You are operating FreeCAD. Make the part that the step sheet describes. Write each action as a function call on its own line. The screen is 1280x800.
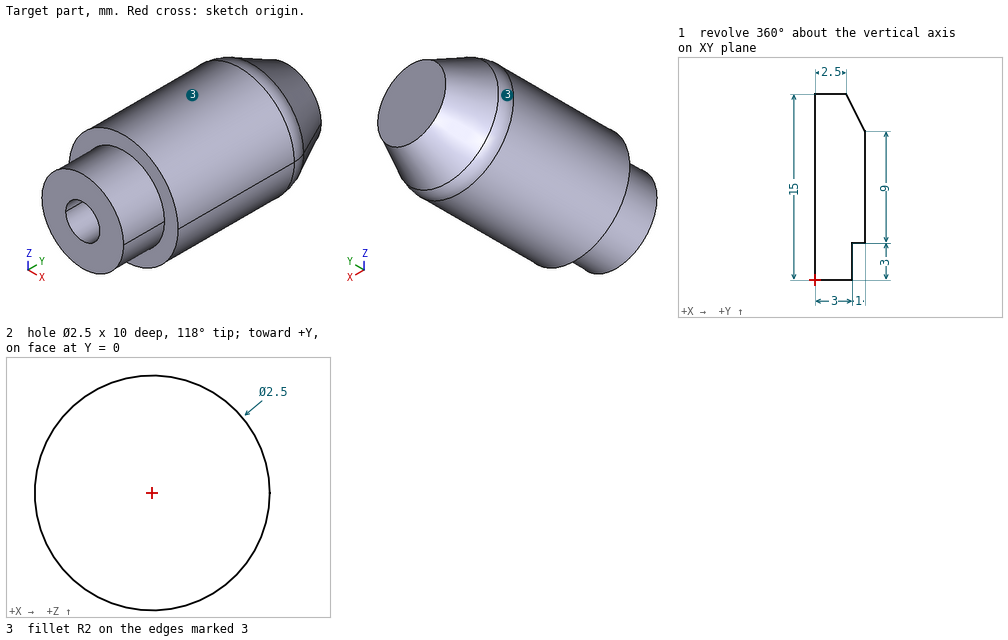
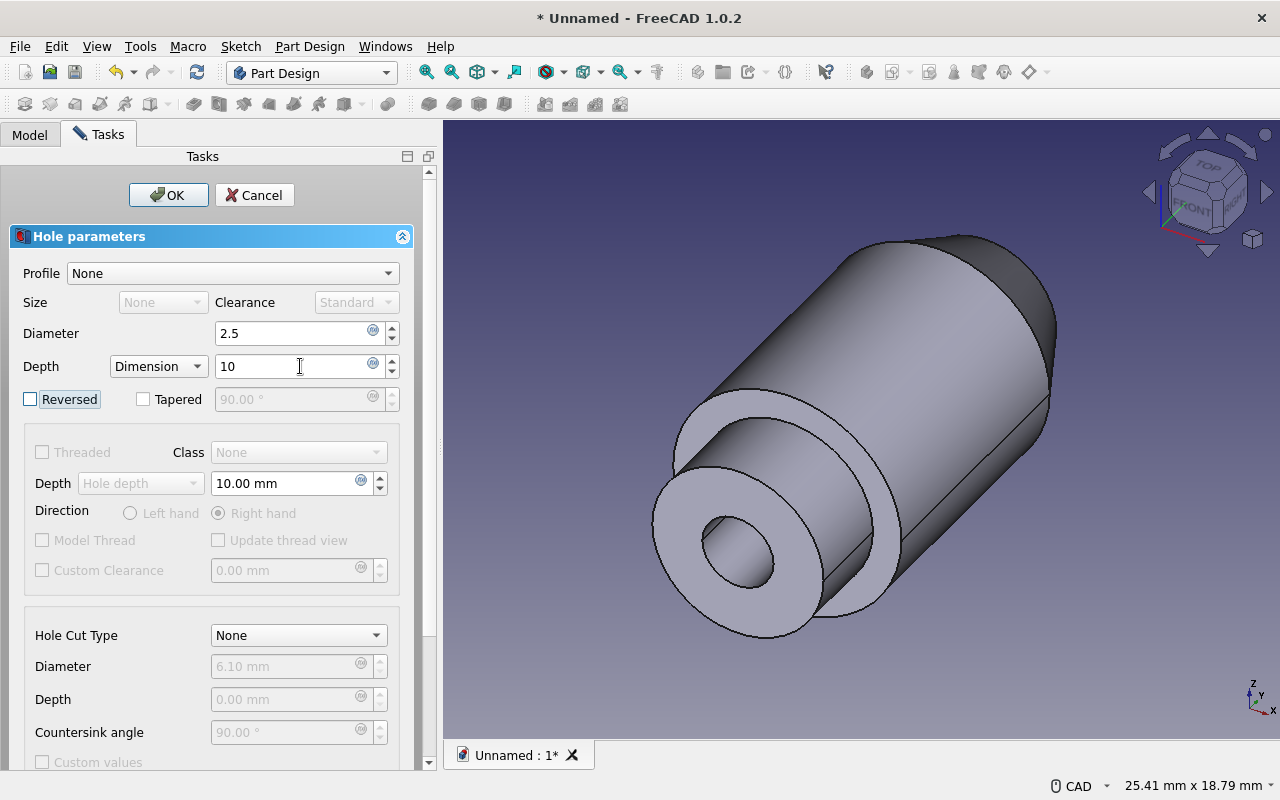
click(169, 195)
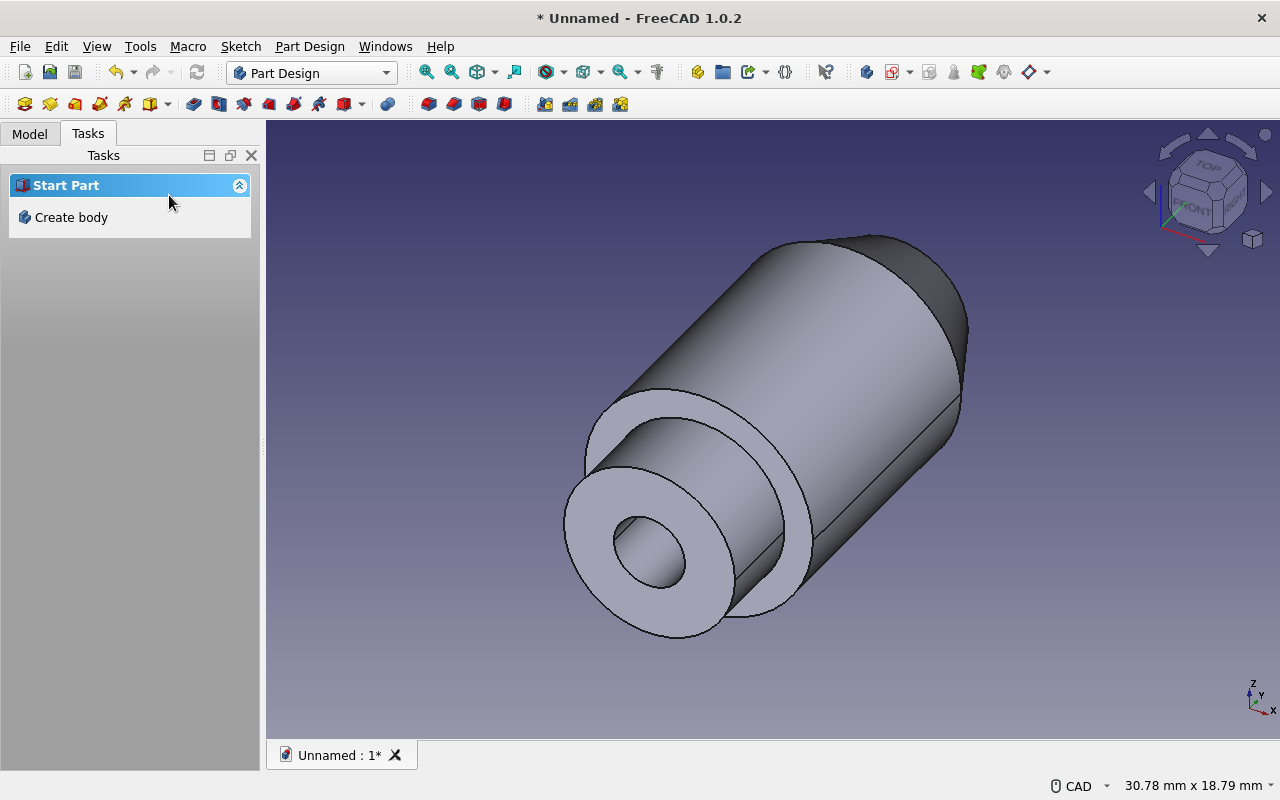
key(0)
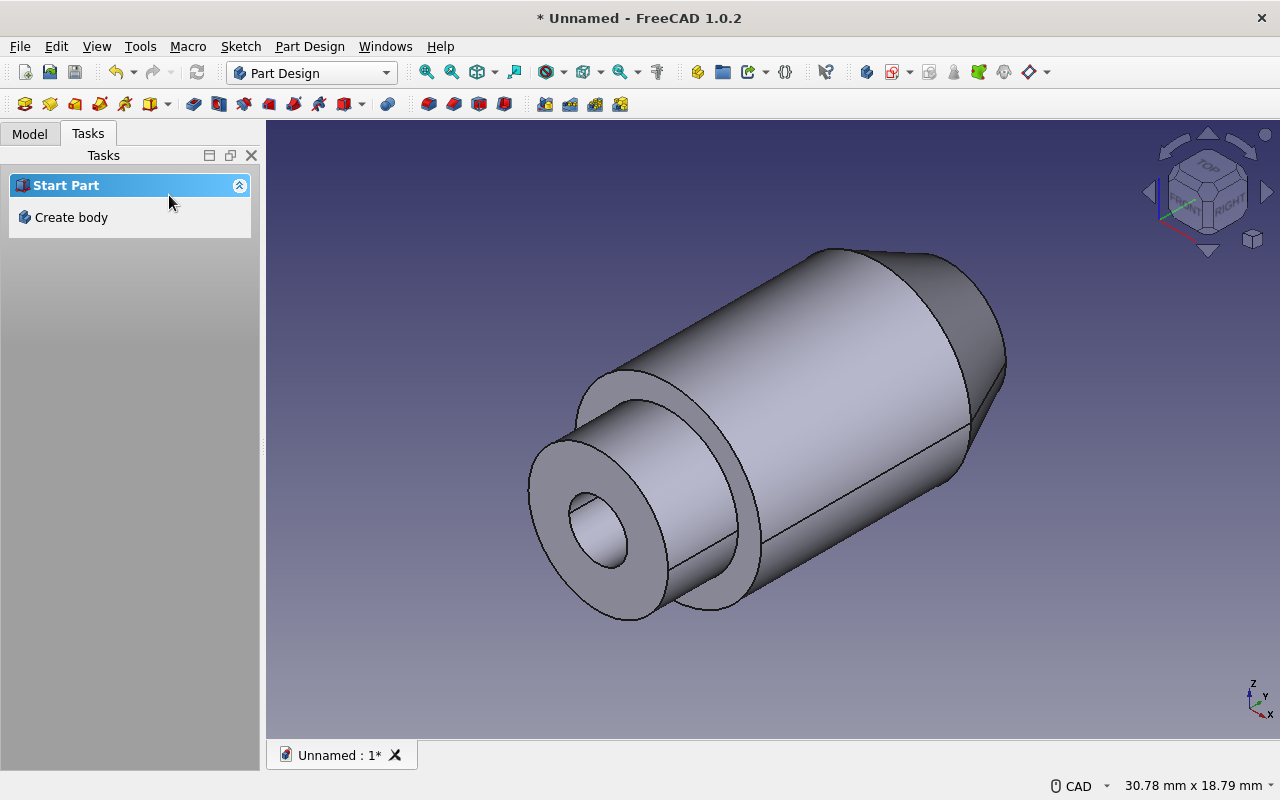
click(849, 249)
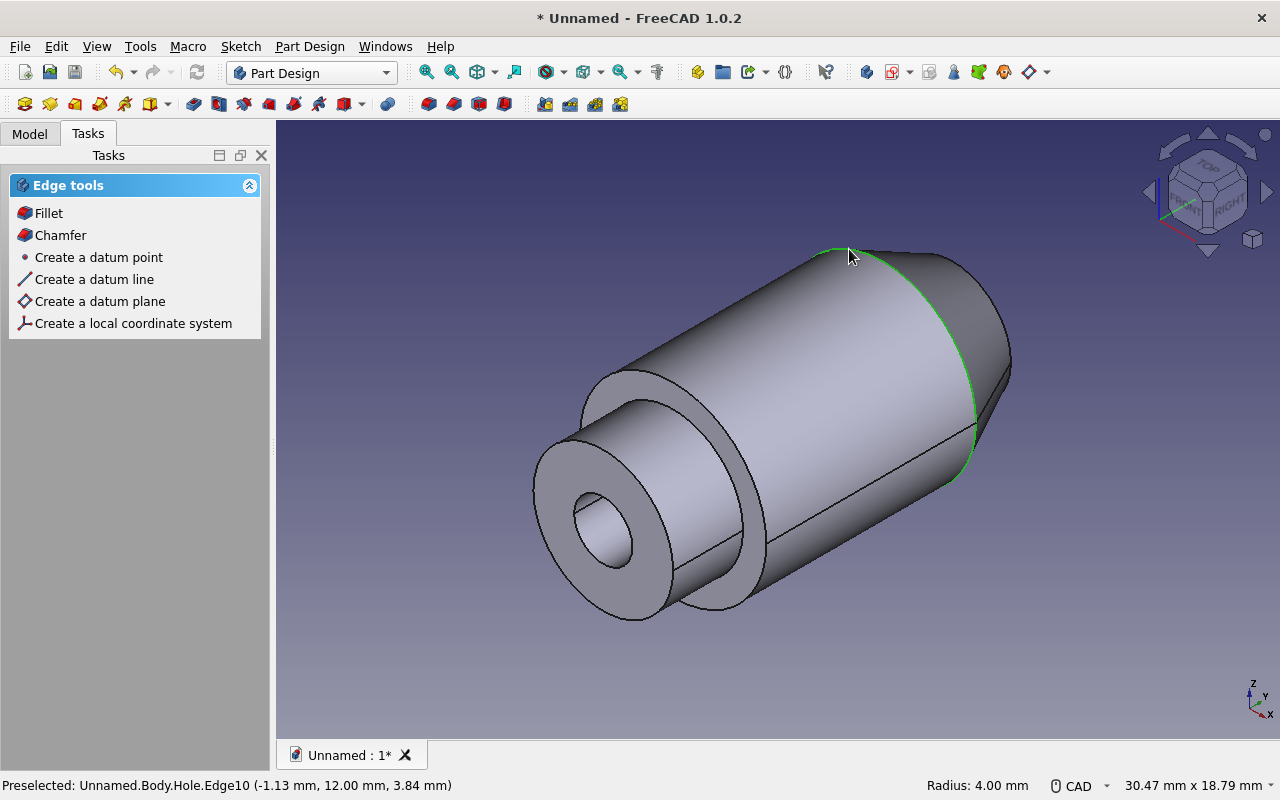
click(429, 104)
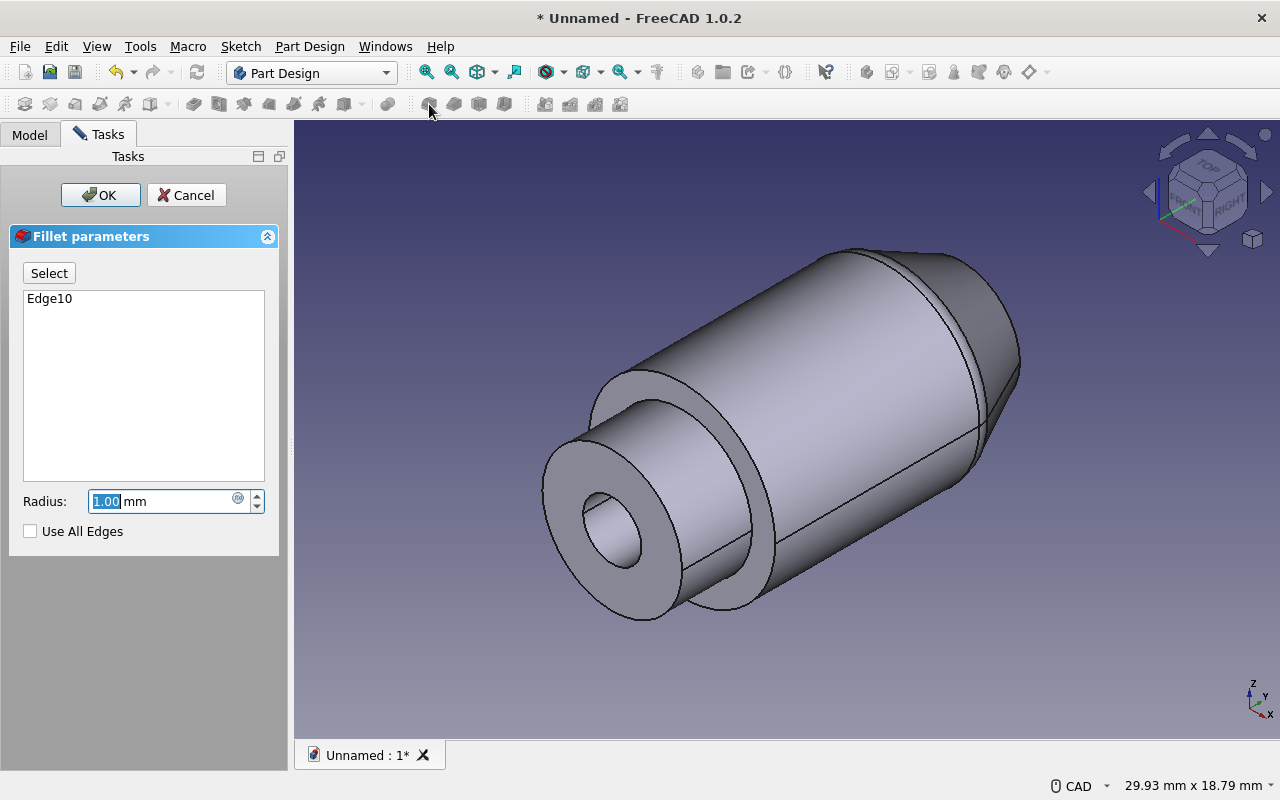
text(2)
key(Tab)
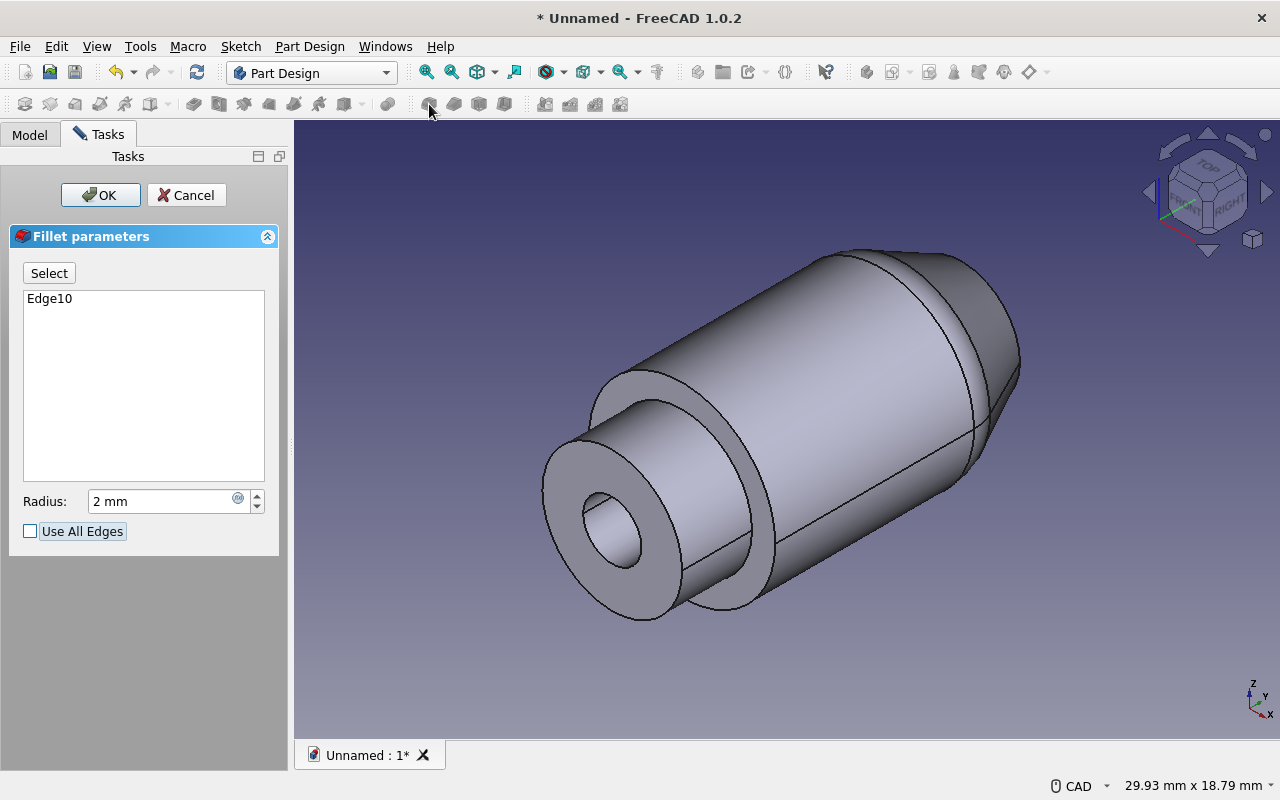
click(101, 195)